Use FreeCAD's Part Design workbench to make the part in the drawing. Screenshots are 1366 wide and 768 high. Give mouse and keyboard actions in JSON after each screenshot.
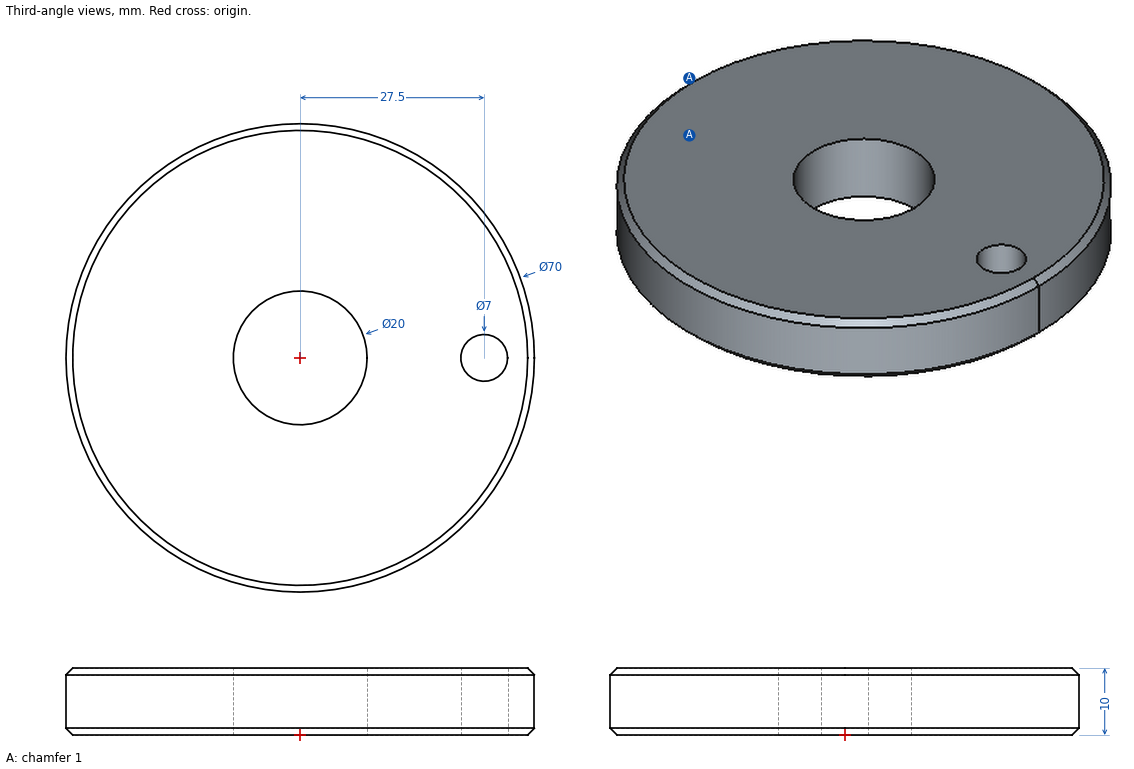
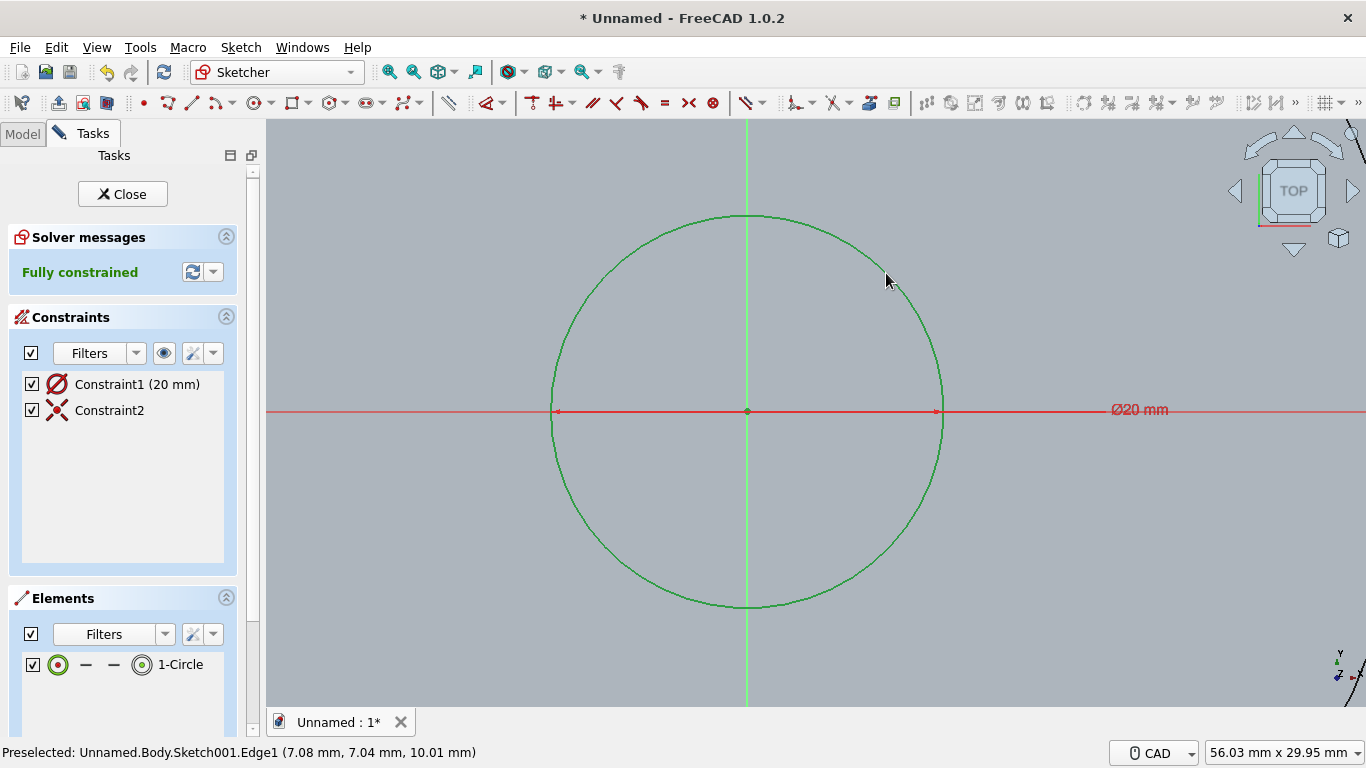
{"action": "left_click", "coordinate": [123, 194]}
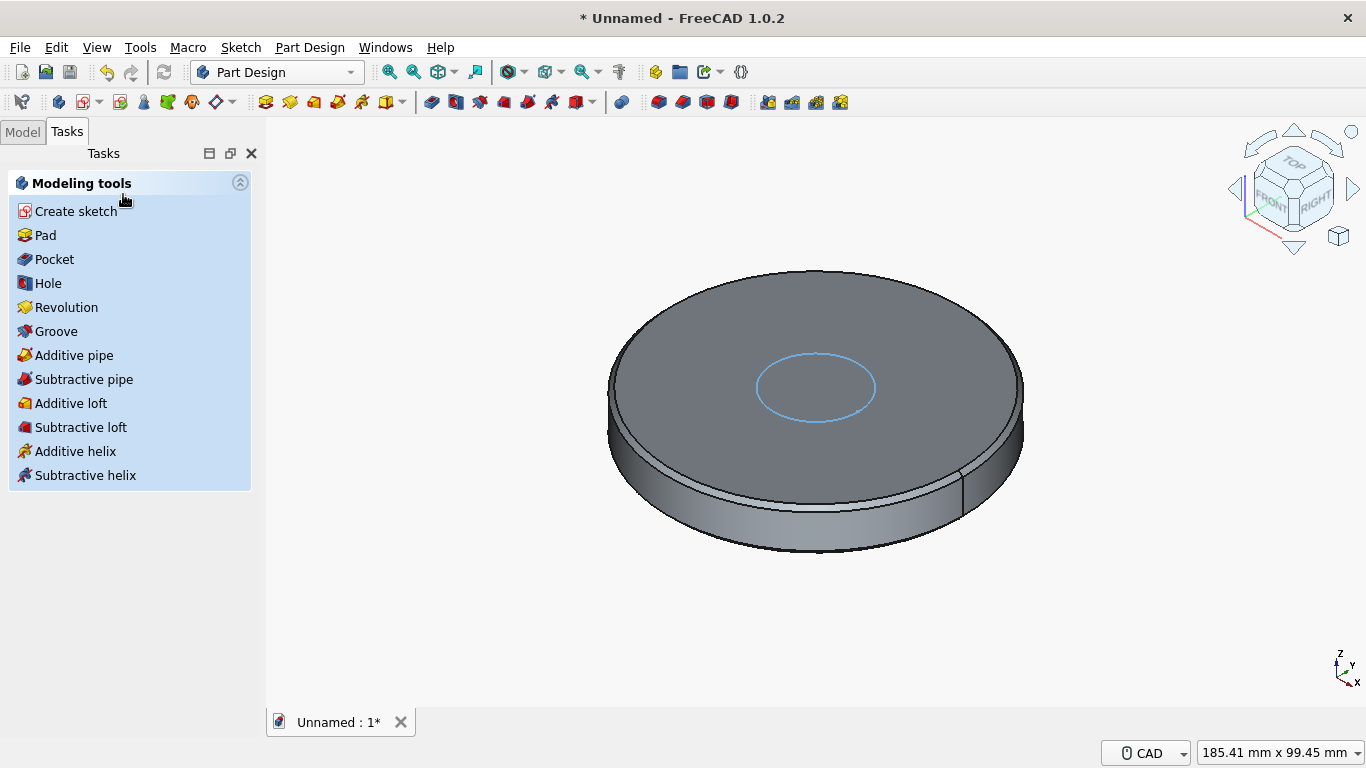
{"action": "left_click", "coordinate": [432, 102]}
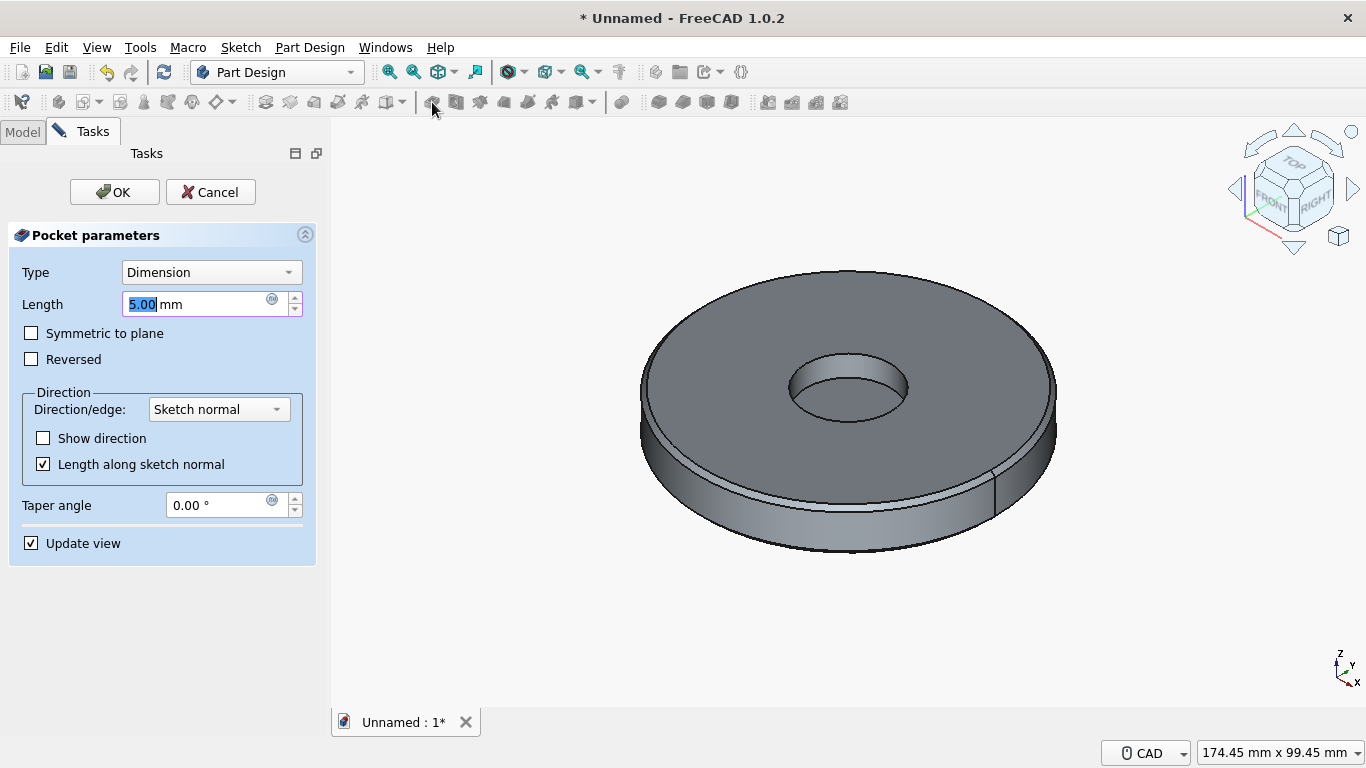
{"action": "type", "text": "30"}
{"action": "key", "text": "Tab"}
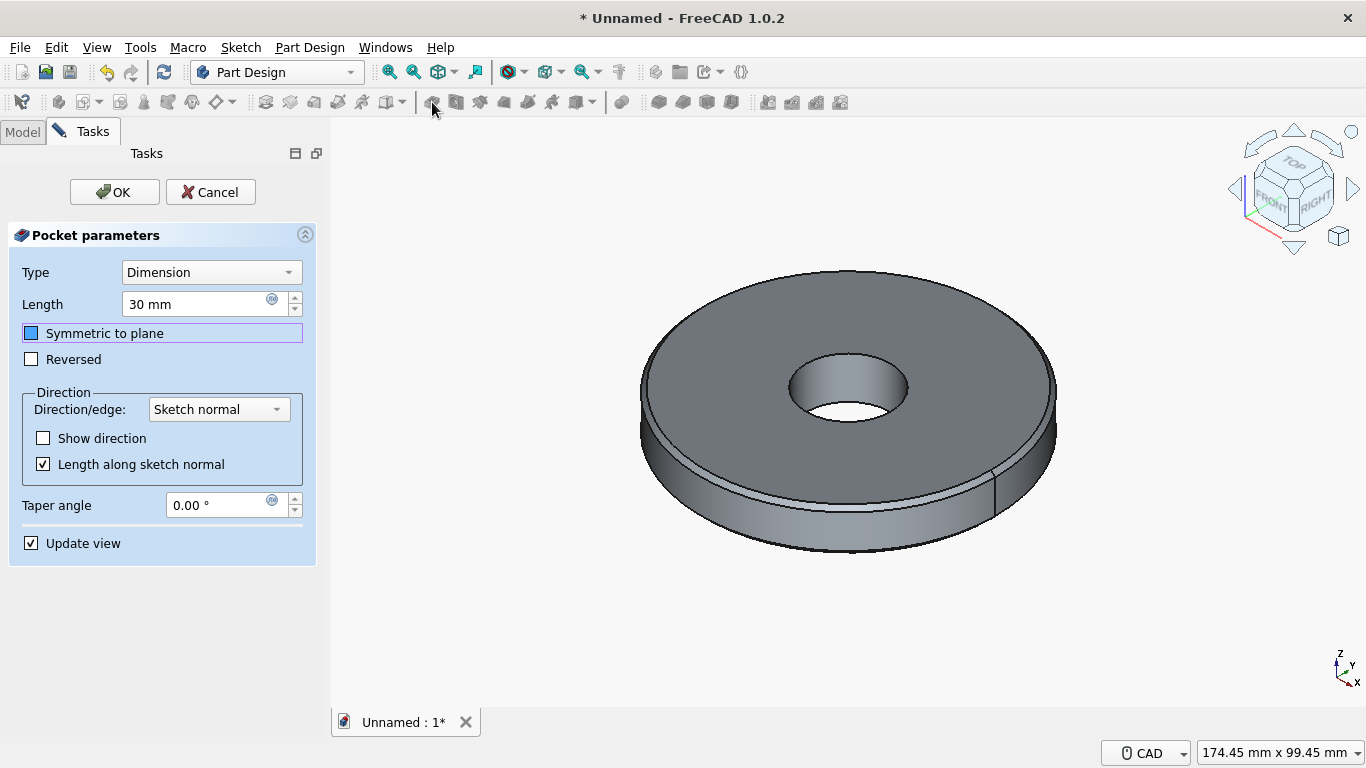
{"action": "left_click", "coordinate": [115, 192]}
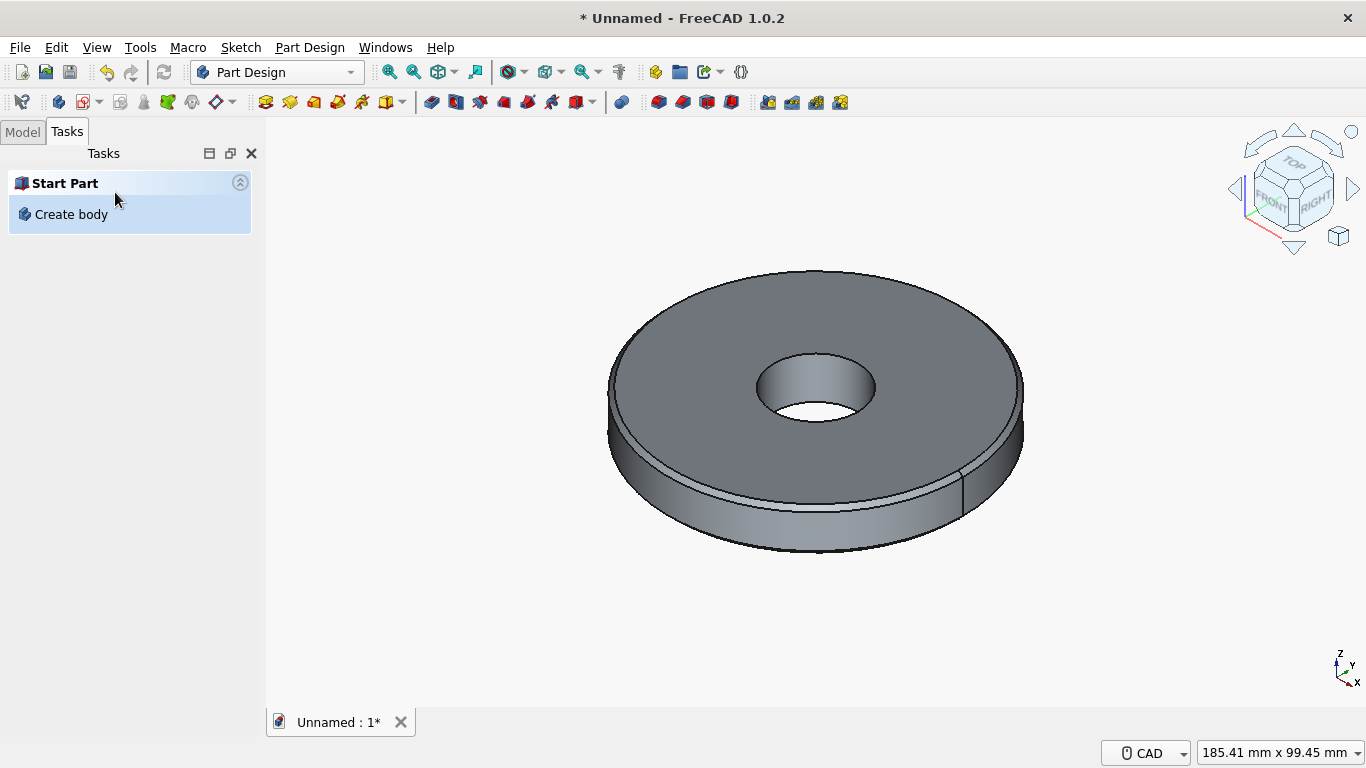
{"action": "left_click", "coordinate": [857, 316]}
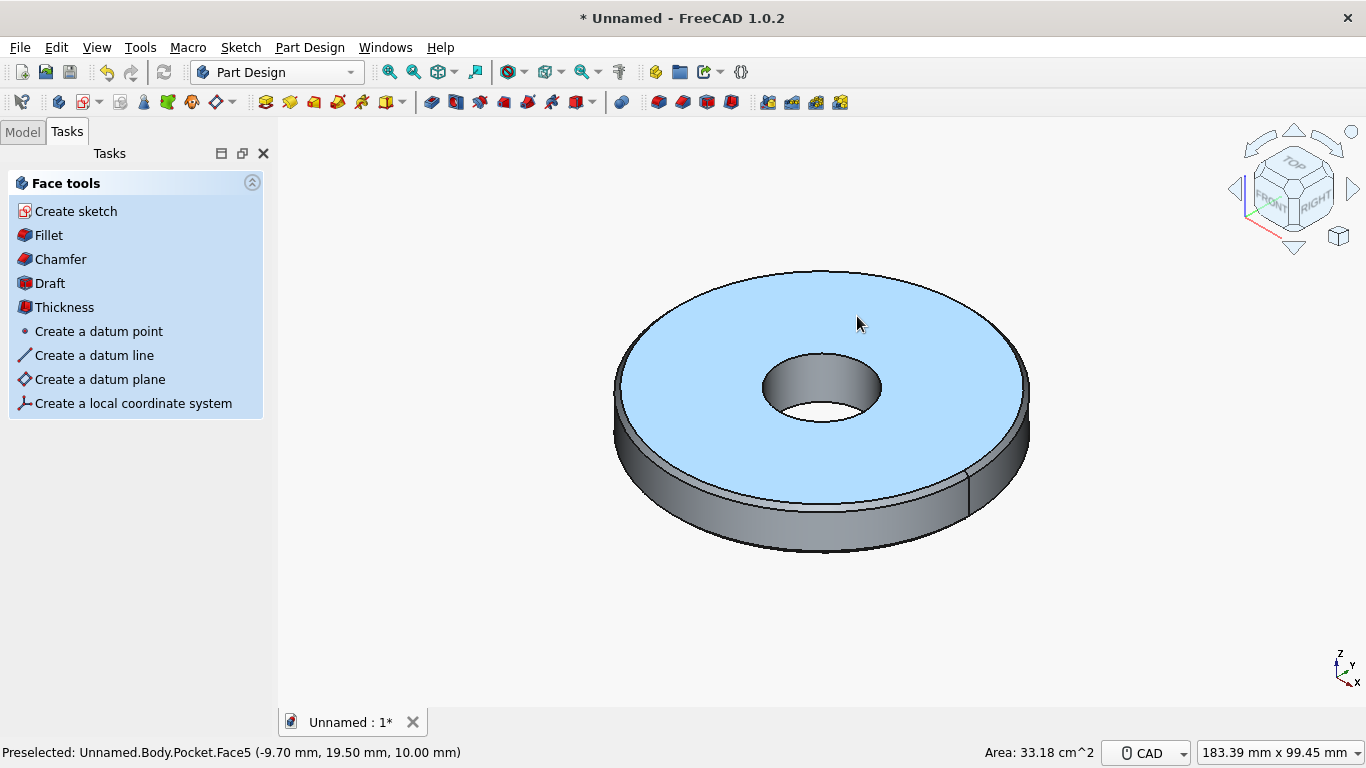
{"action": "left_click", "coordinate": [84, 102]}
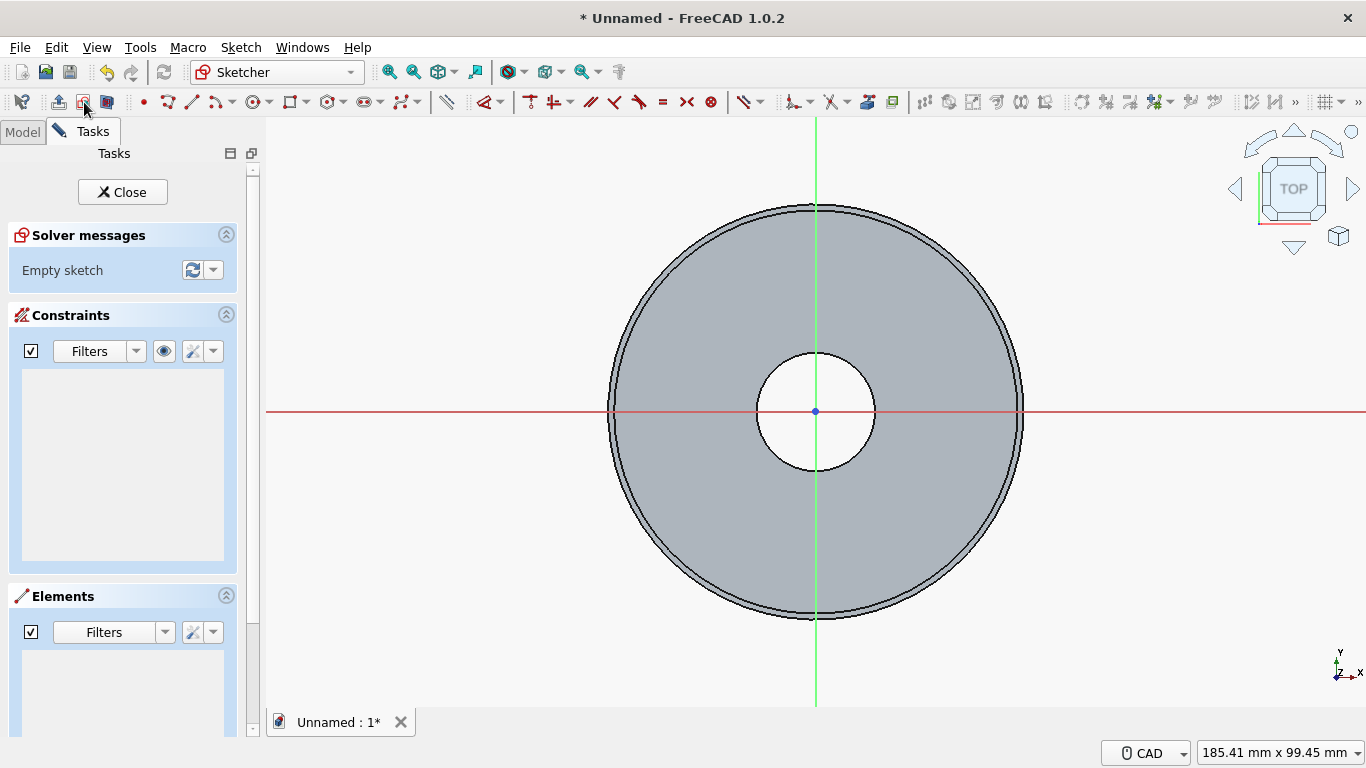
{"action": "scroll", "coordinate": [1008, 412], "scroll_direction": "up", "scroll_amount": 11}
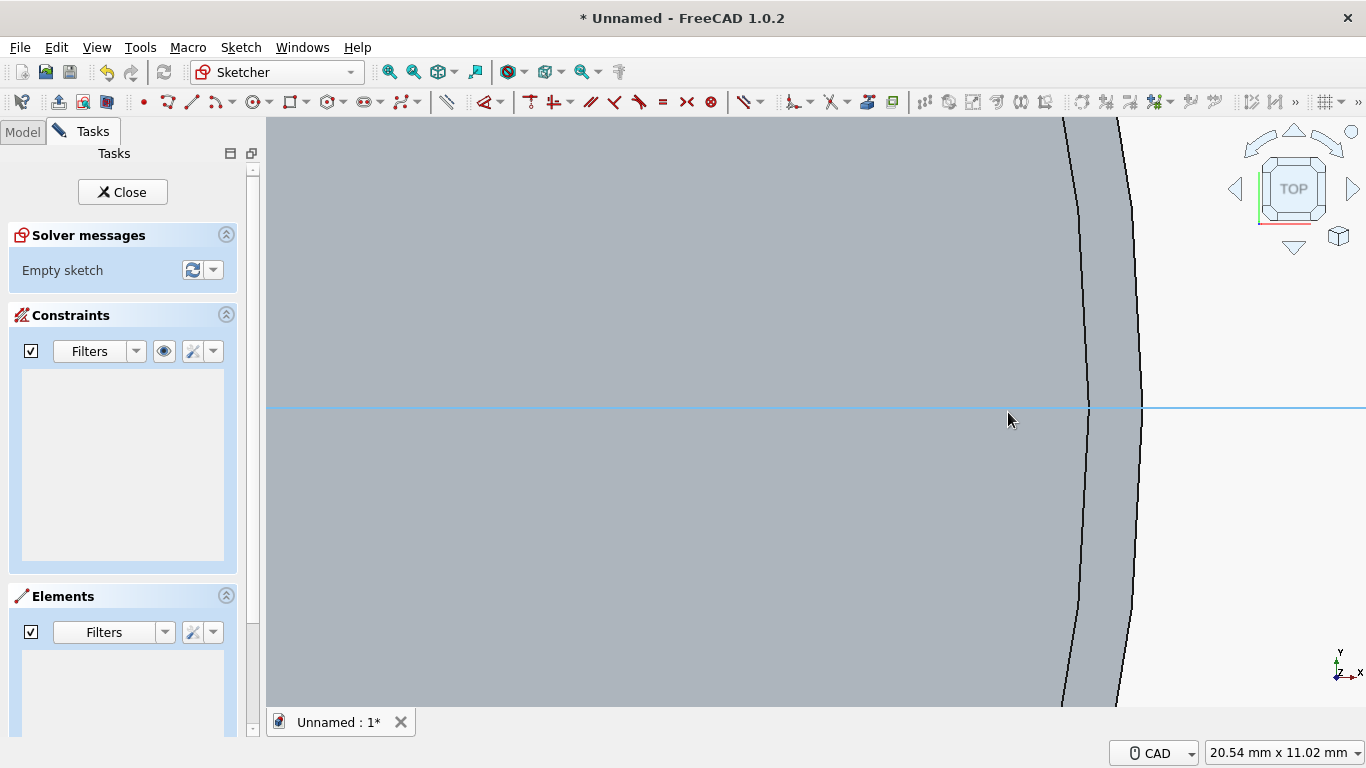
{"action": "left_click", "coordinate": [254, 102]}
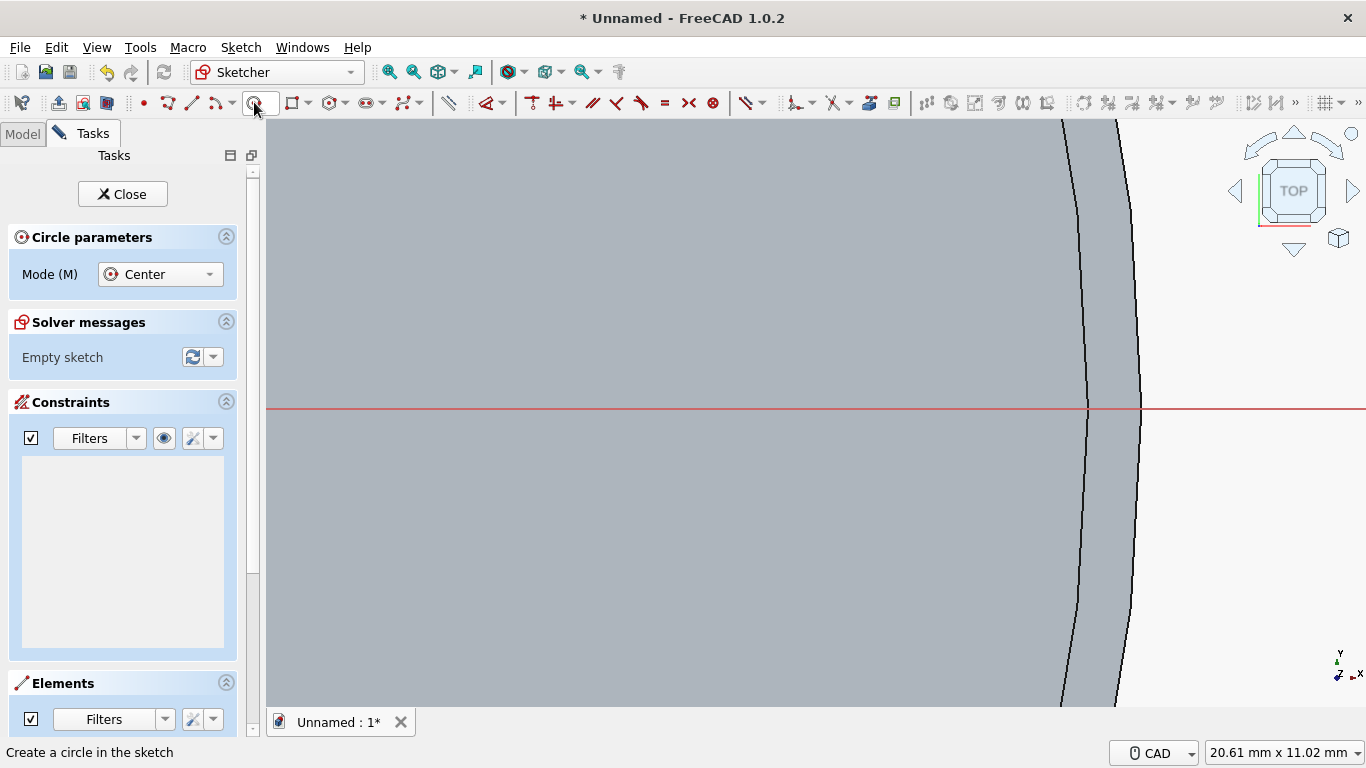
{"action": "left_click", "coordinate": [741, 409]}
{"action": "mouse_move", "coordinate": [873, 277]}